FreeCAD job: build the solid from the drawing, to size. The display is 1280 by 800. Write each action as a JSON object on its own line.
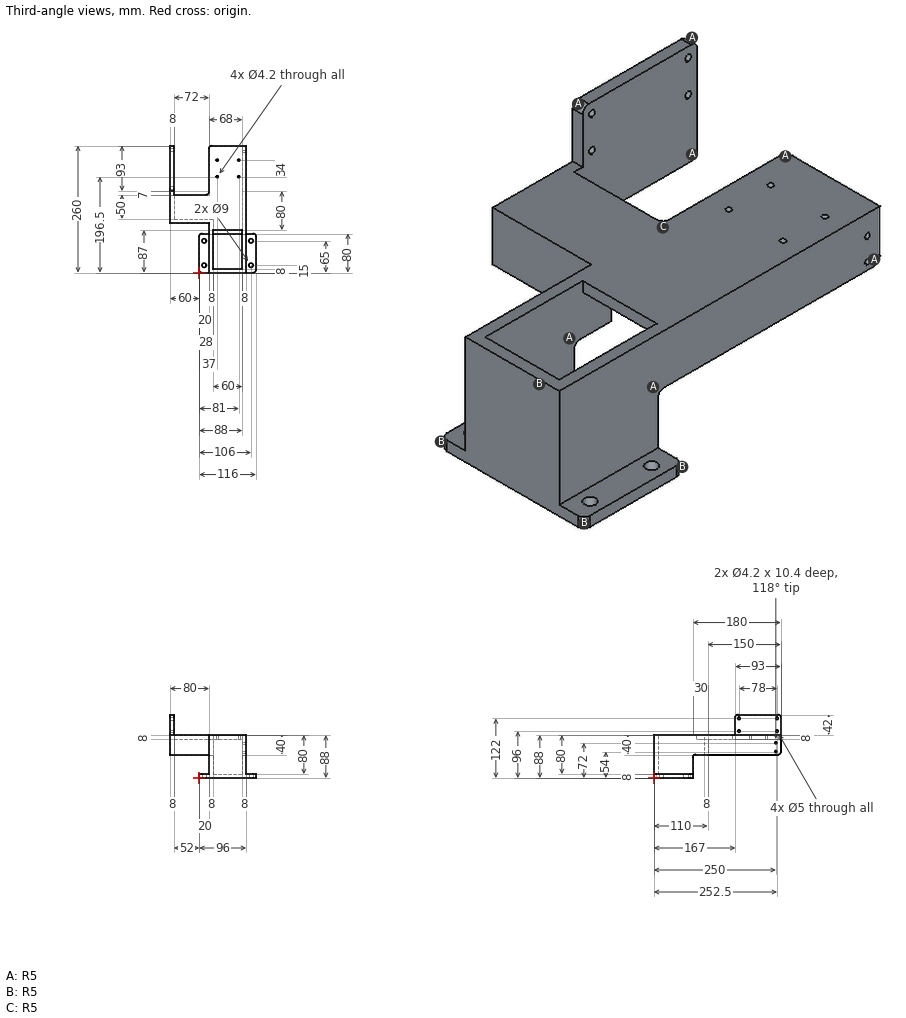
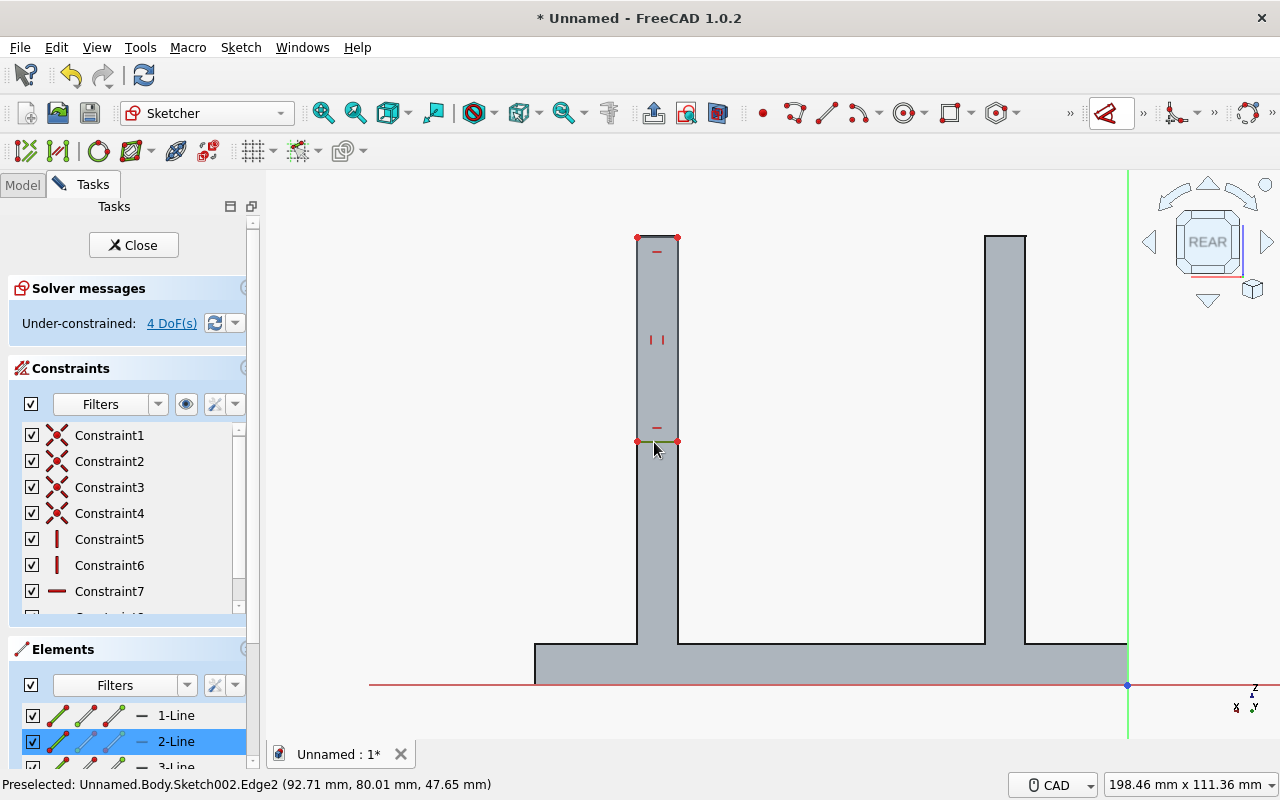
{"action": "left_click", "coordinate": [1128, 114]}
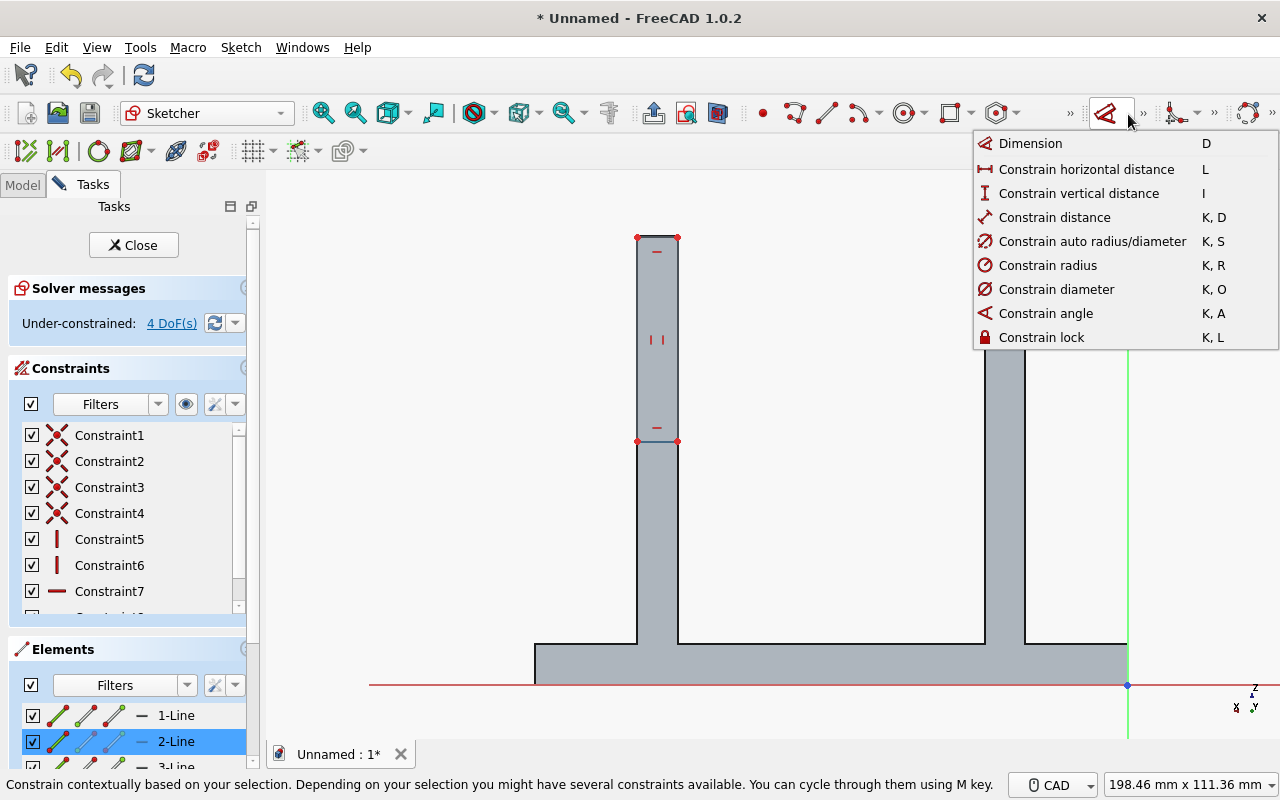
{"action": "left_click", "coordinate": [1126, 169]}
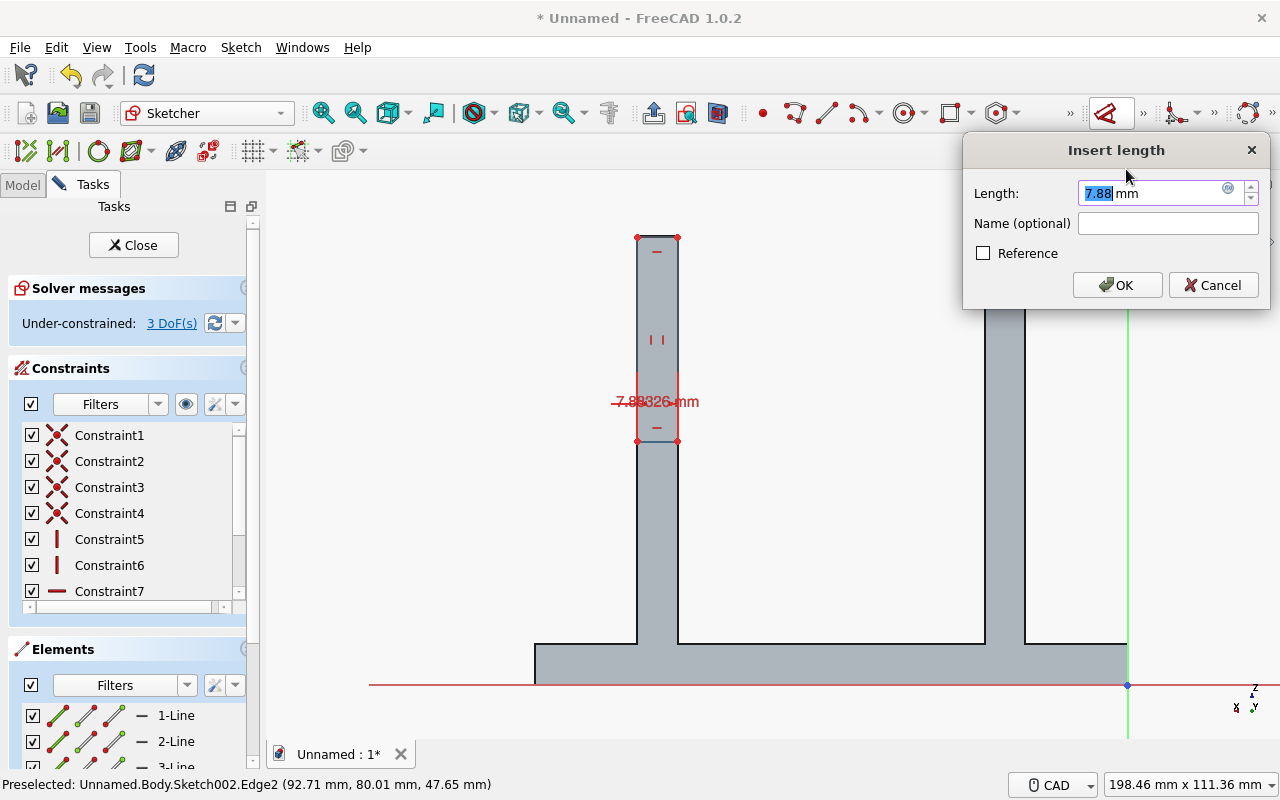
{"action": "type", "text": "8"}
{"action": "key", "text": "Return"}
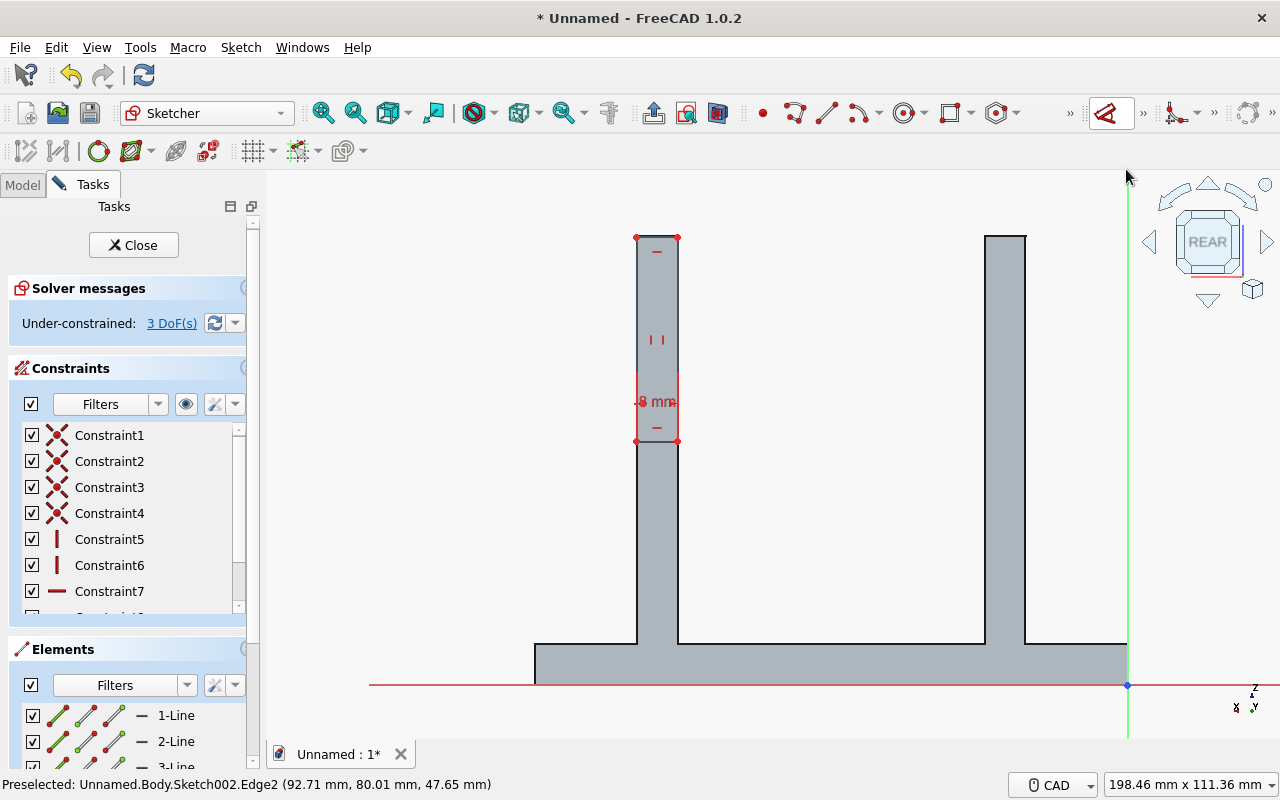
{"action": "left_click", "coordinate": [637, 299]}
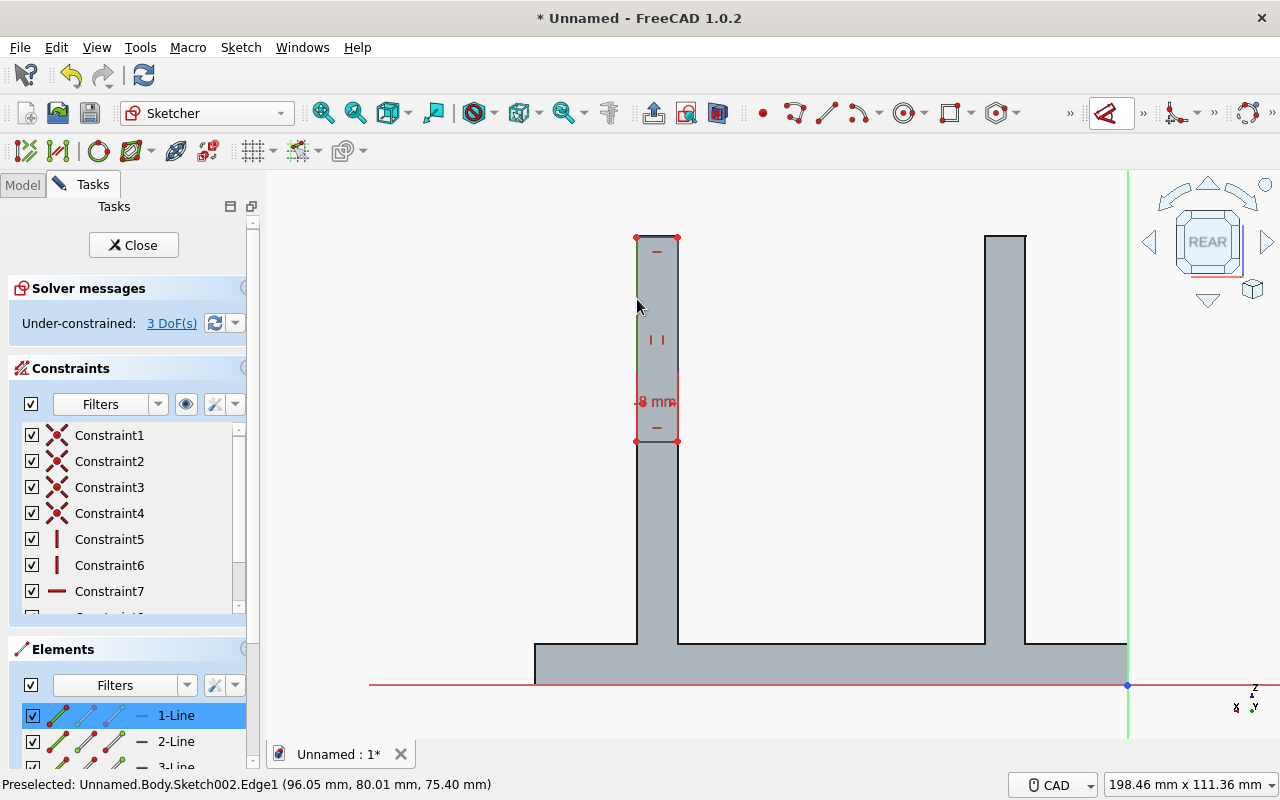
{"action": "left_click", "coordinate": [1128, 114]}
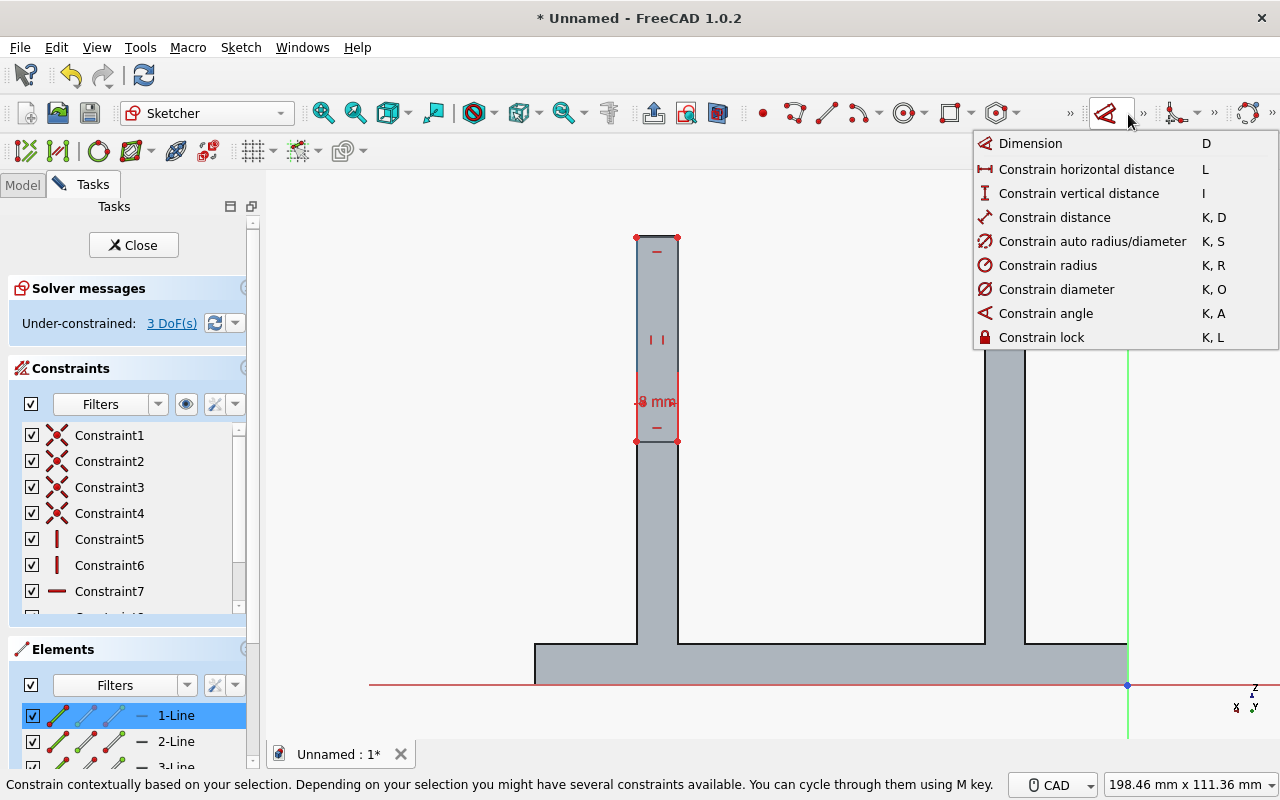
{"action": "left_click", "coordinate": [1126, 193]}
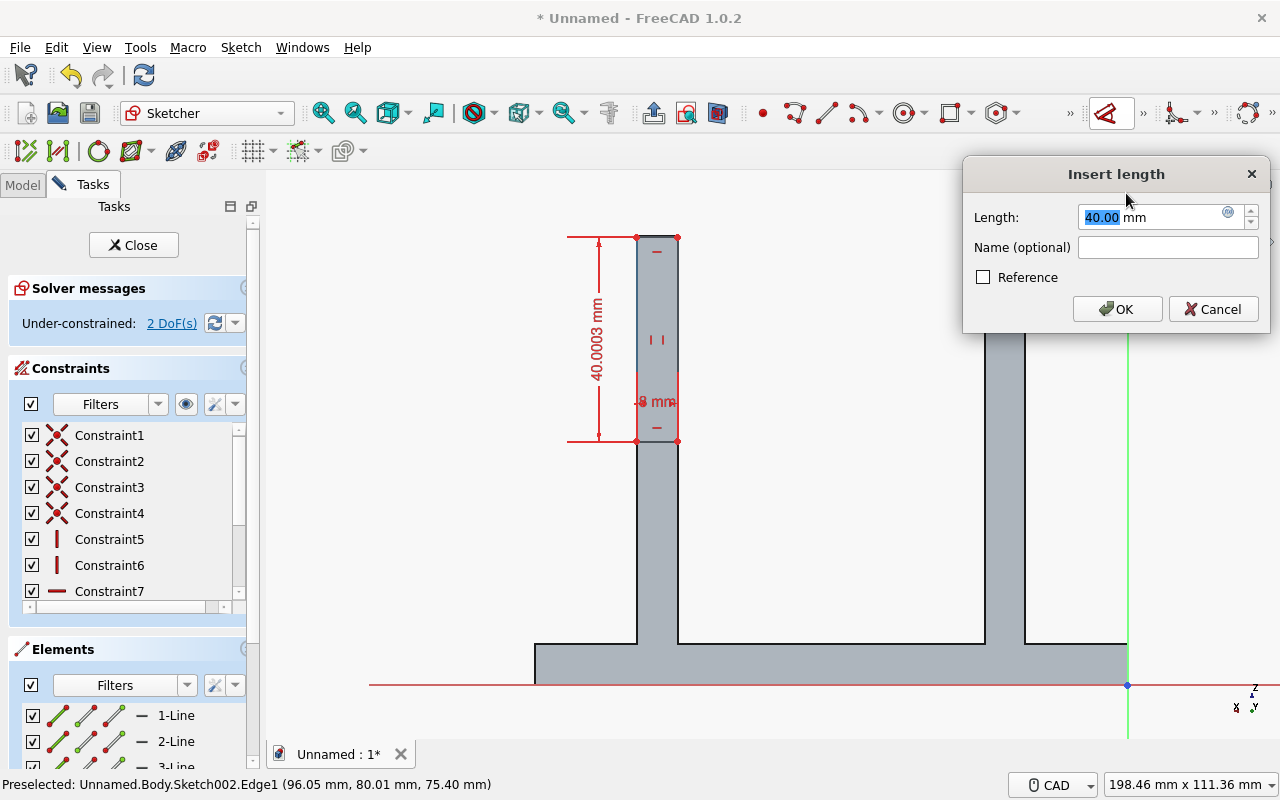
{"action": "type", "text": "40"}
{"action": "key", "text": "Return"}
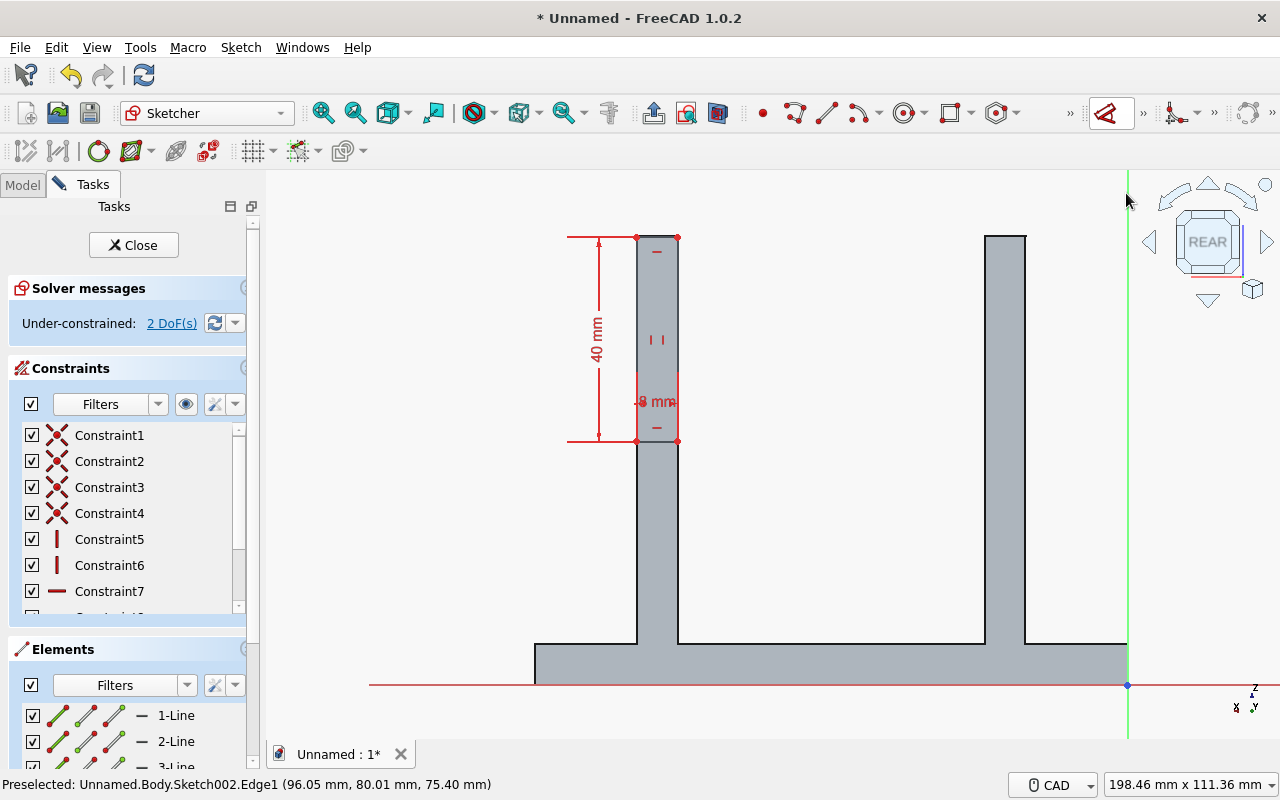
{"action": "left_click", "coordinate": [637, 237]}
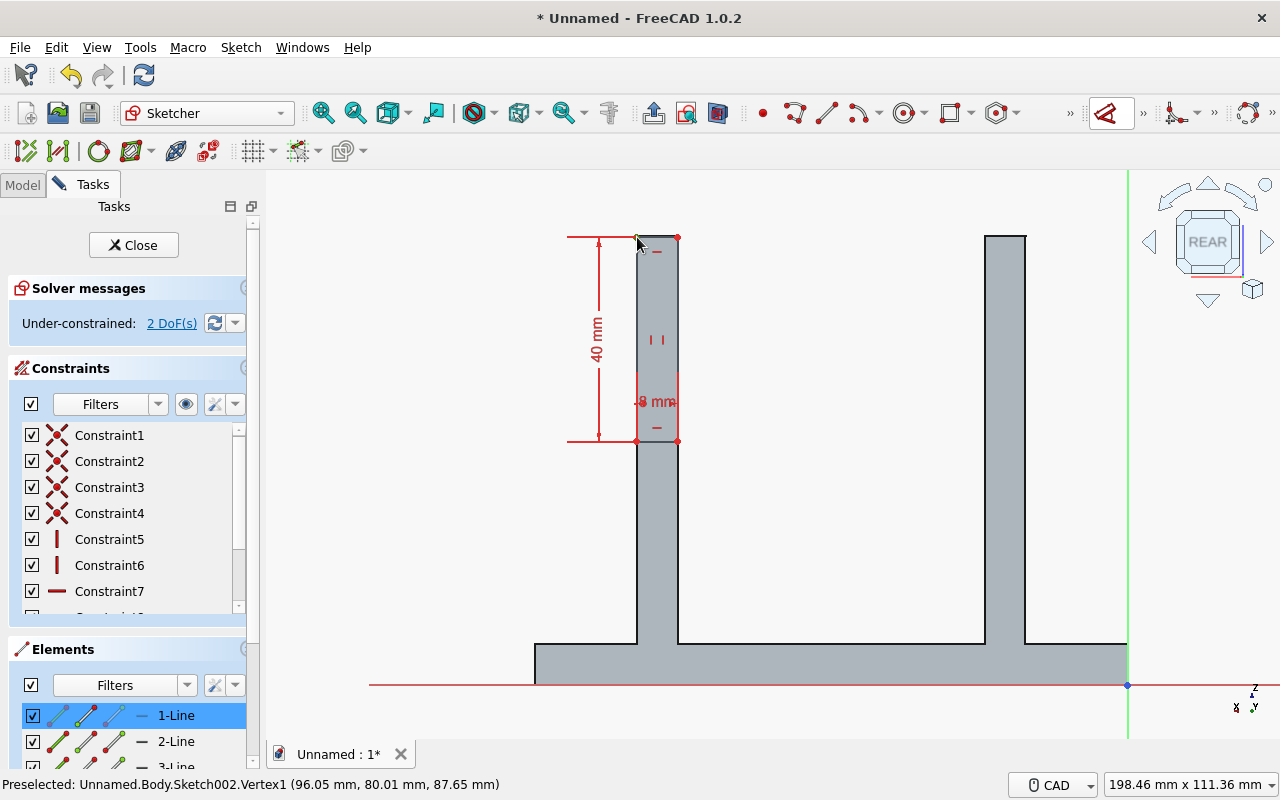
{"action": "left_click", "coordinate": [1128, 114]}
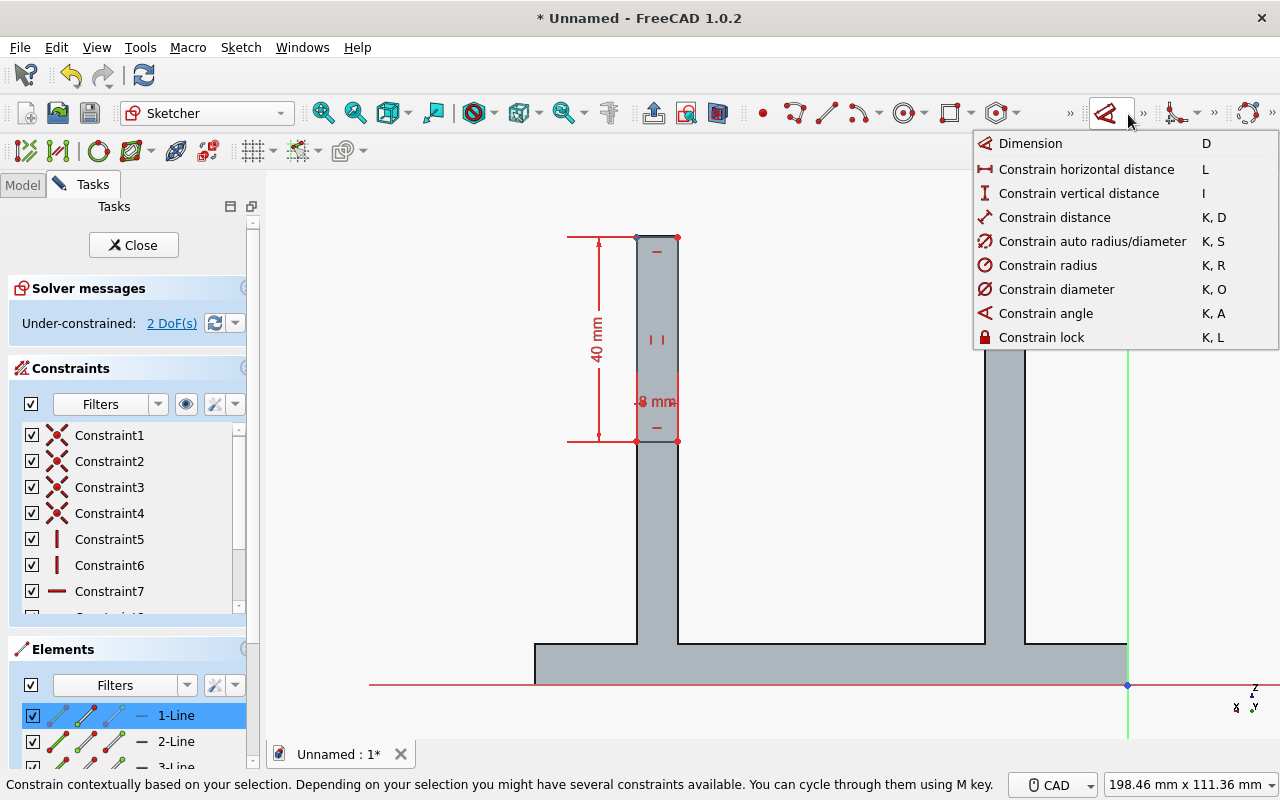
{"action": "left_click", "coordinate": [1126, 169]}